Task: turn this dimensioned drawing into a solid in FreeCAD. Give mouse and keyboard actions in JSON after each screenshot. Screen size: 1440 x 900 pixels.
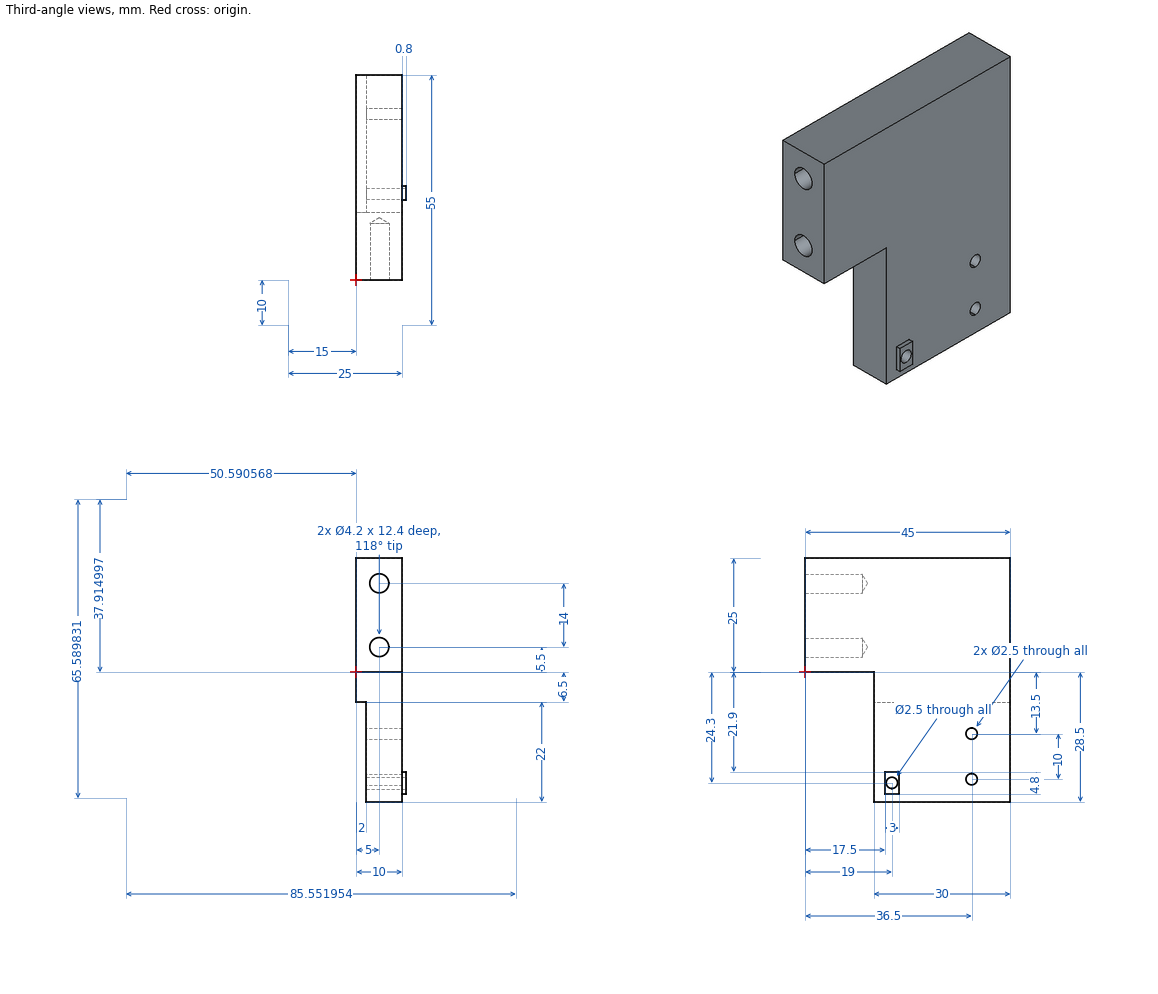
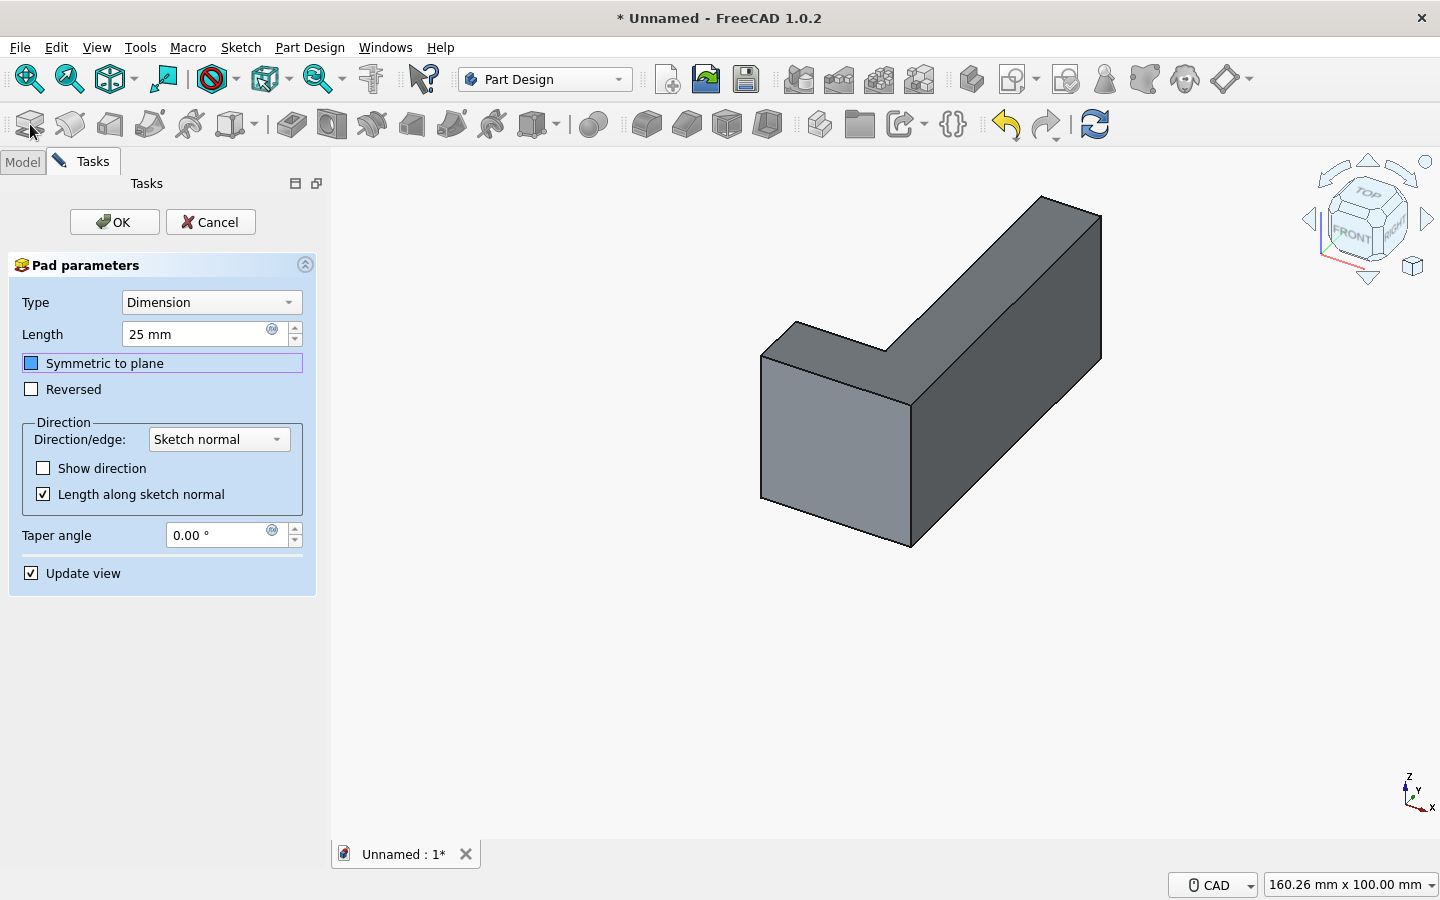
{"action": "left_click", "coordinate": [115, 222]}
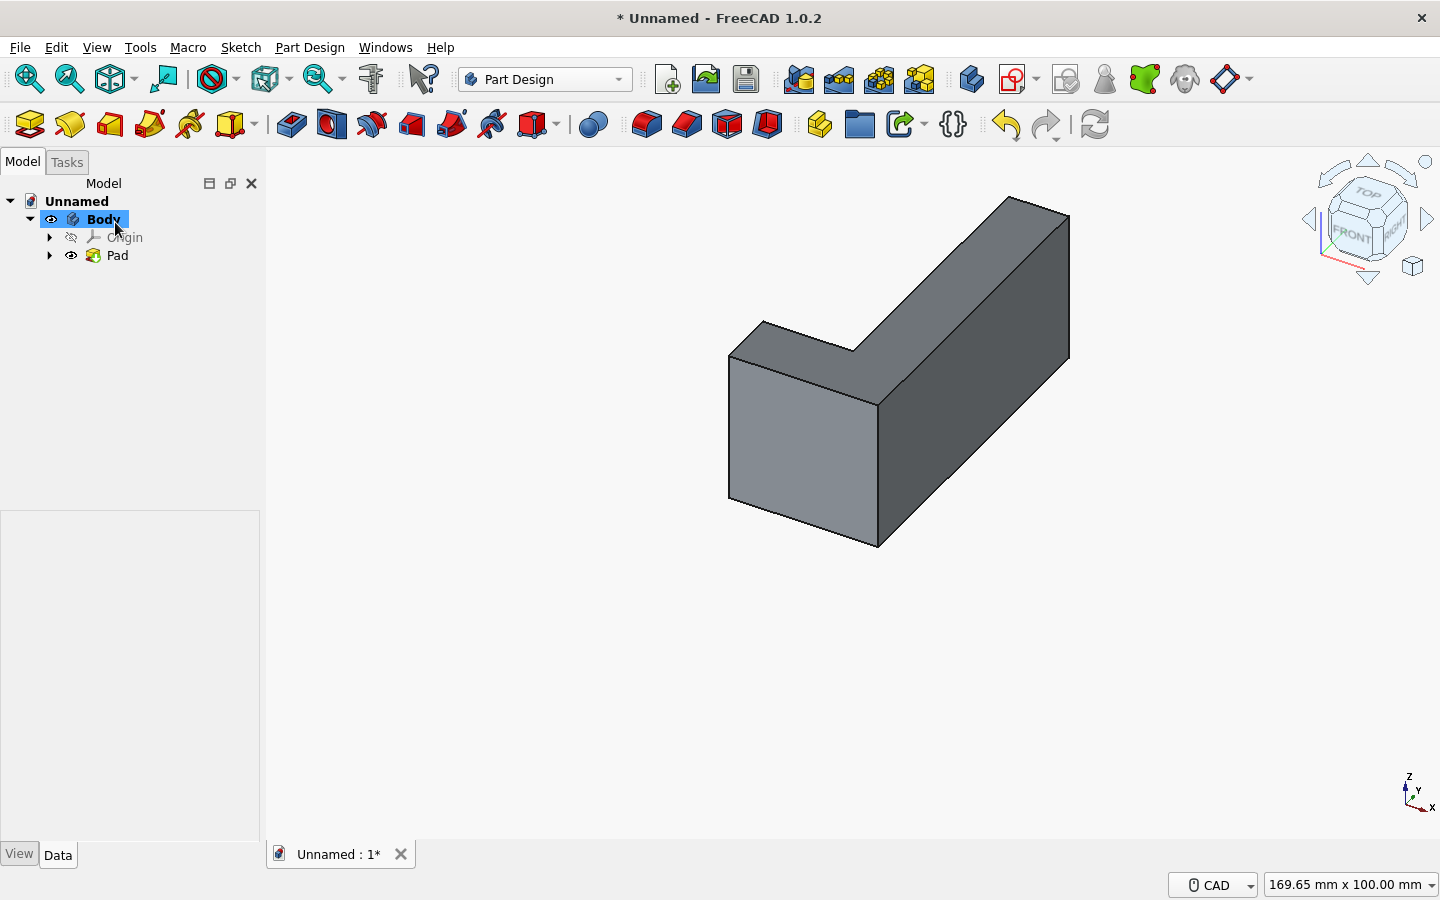
{"action": "key", "text": "6"}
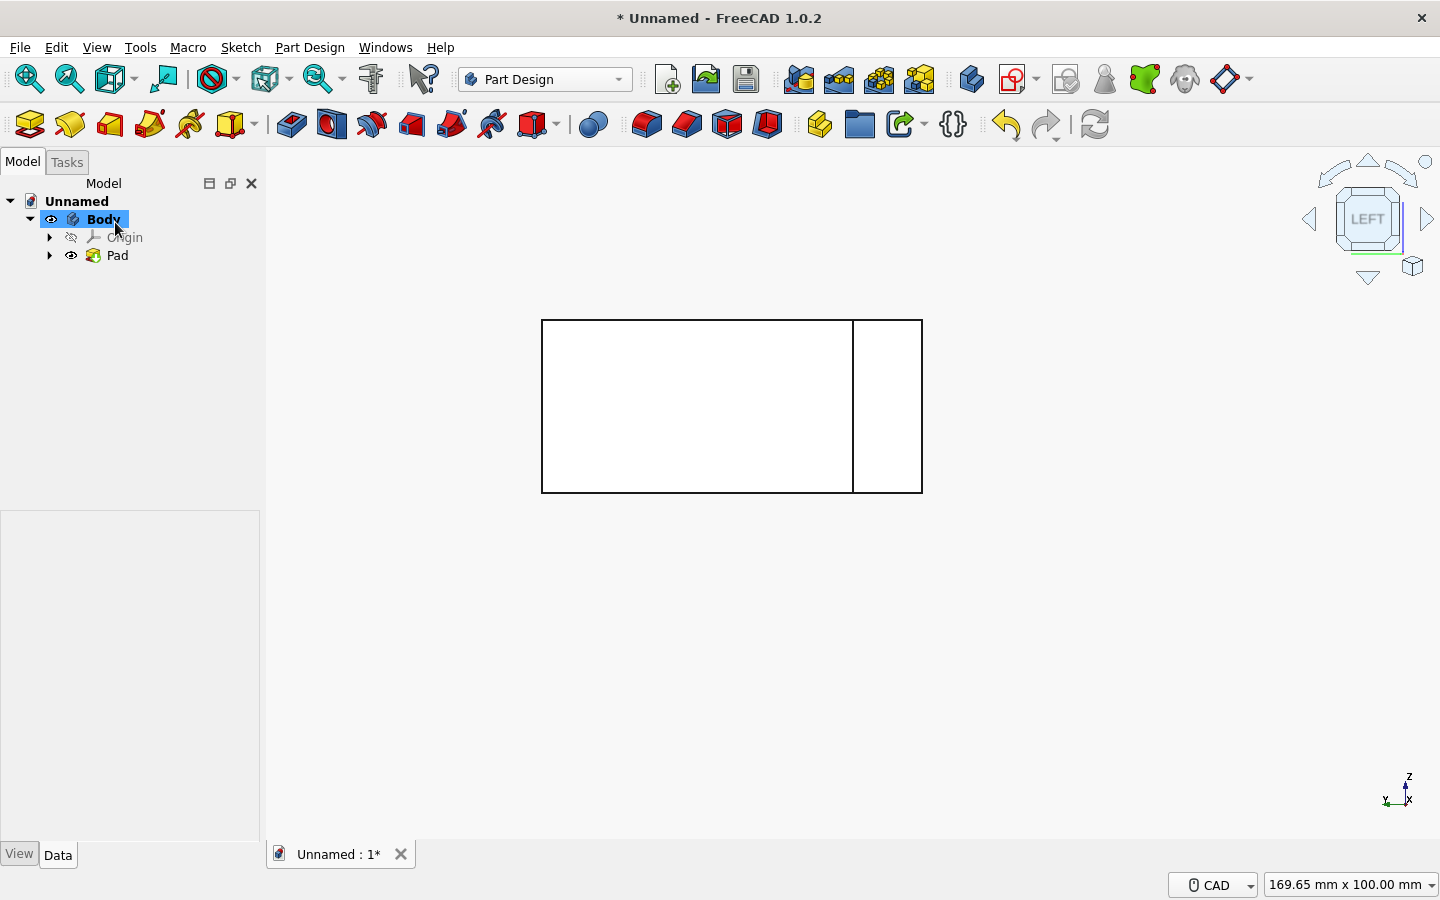
{"action": "key", "text": "v f"}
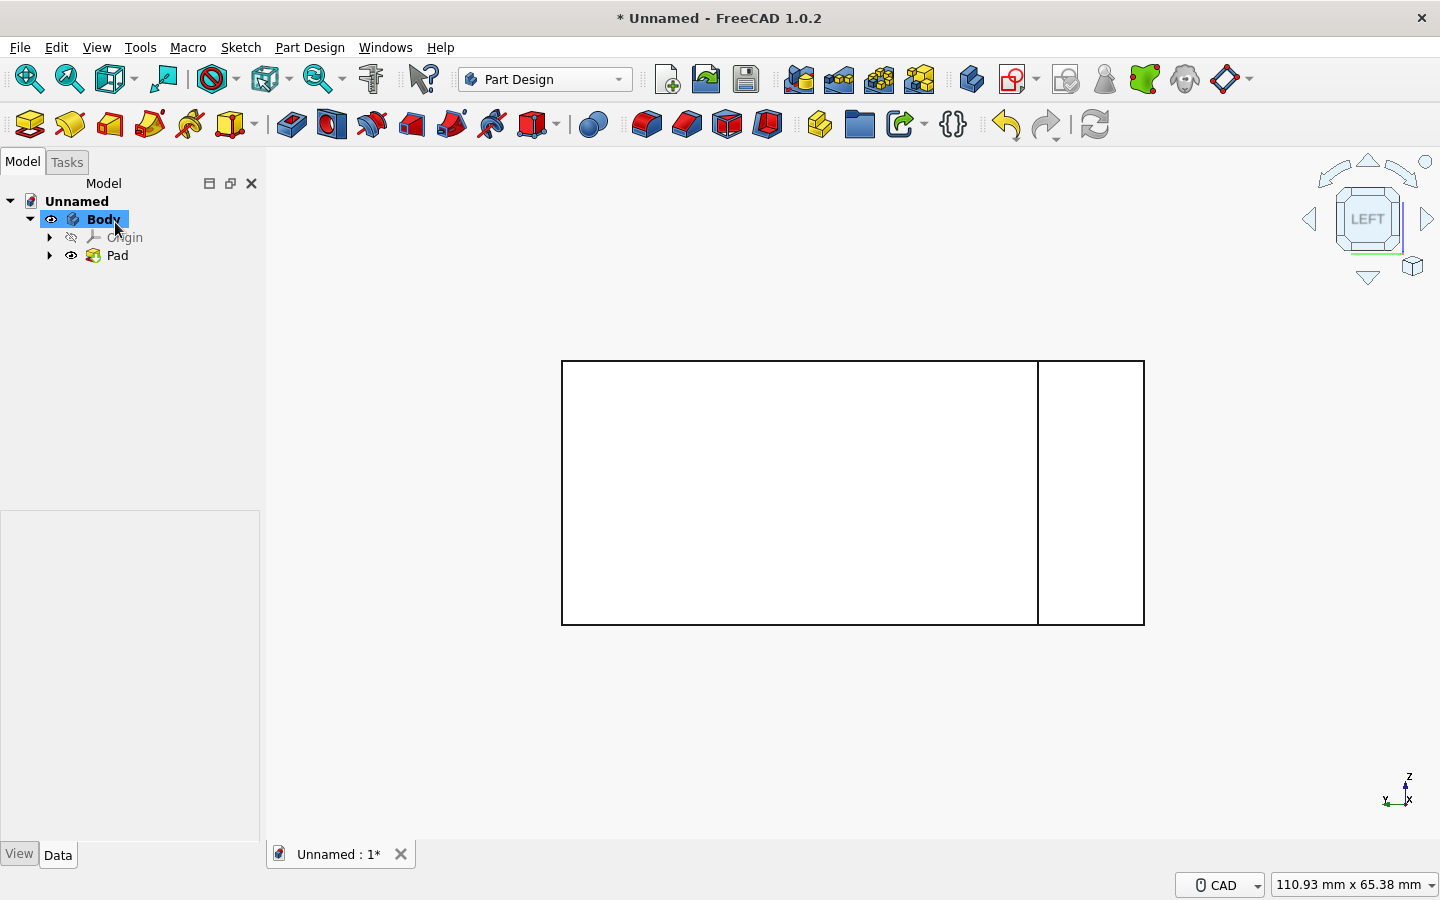
{"action": "left_click", "coordinate": [732, 492]}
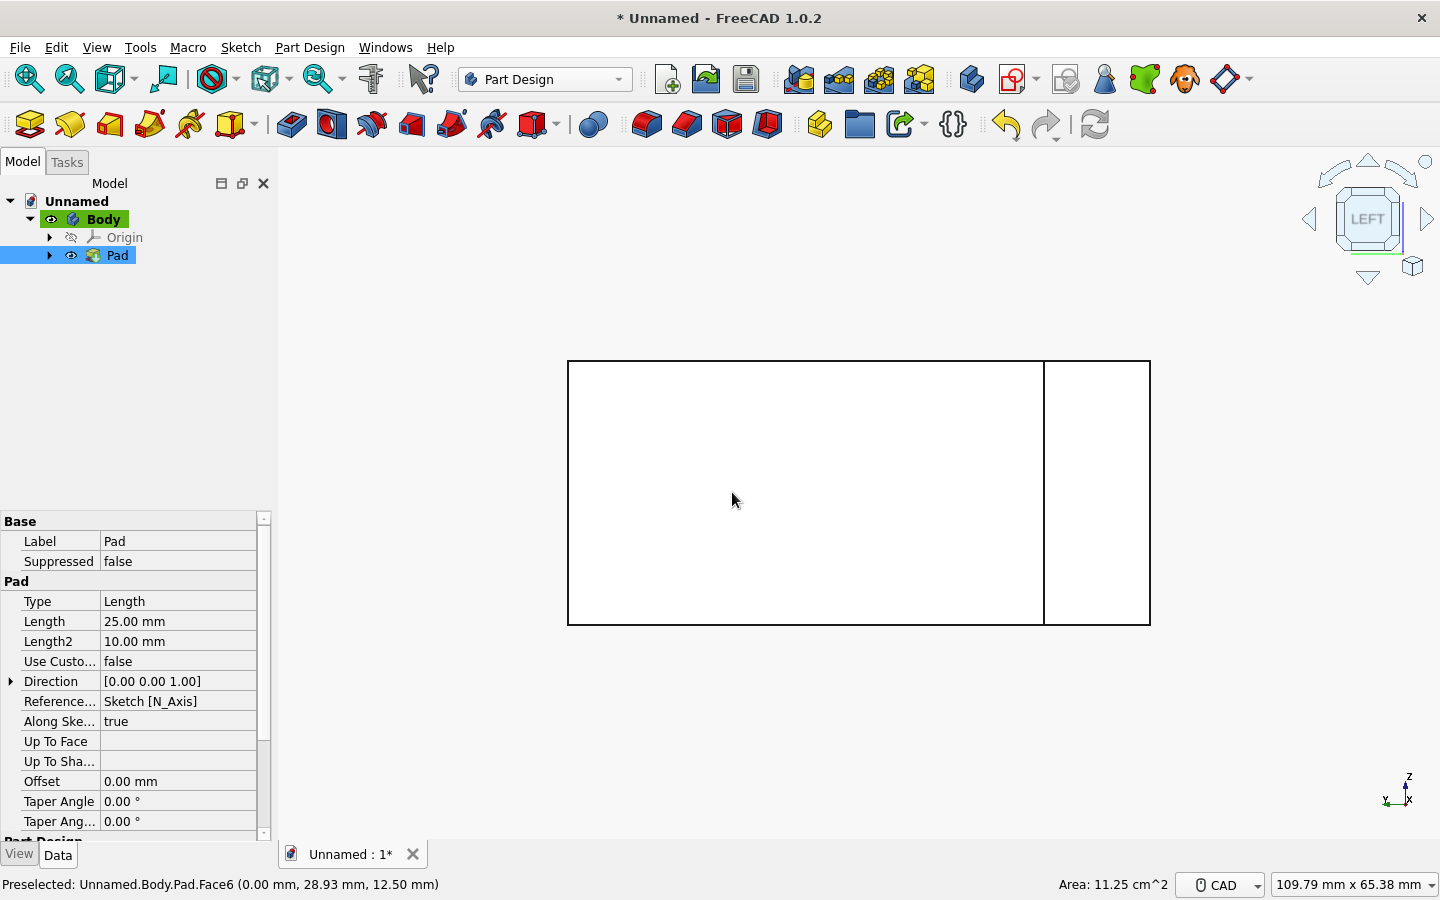
{"action": "left_click", "coordinate": [1012, 80]}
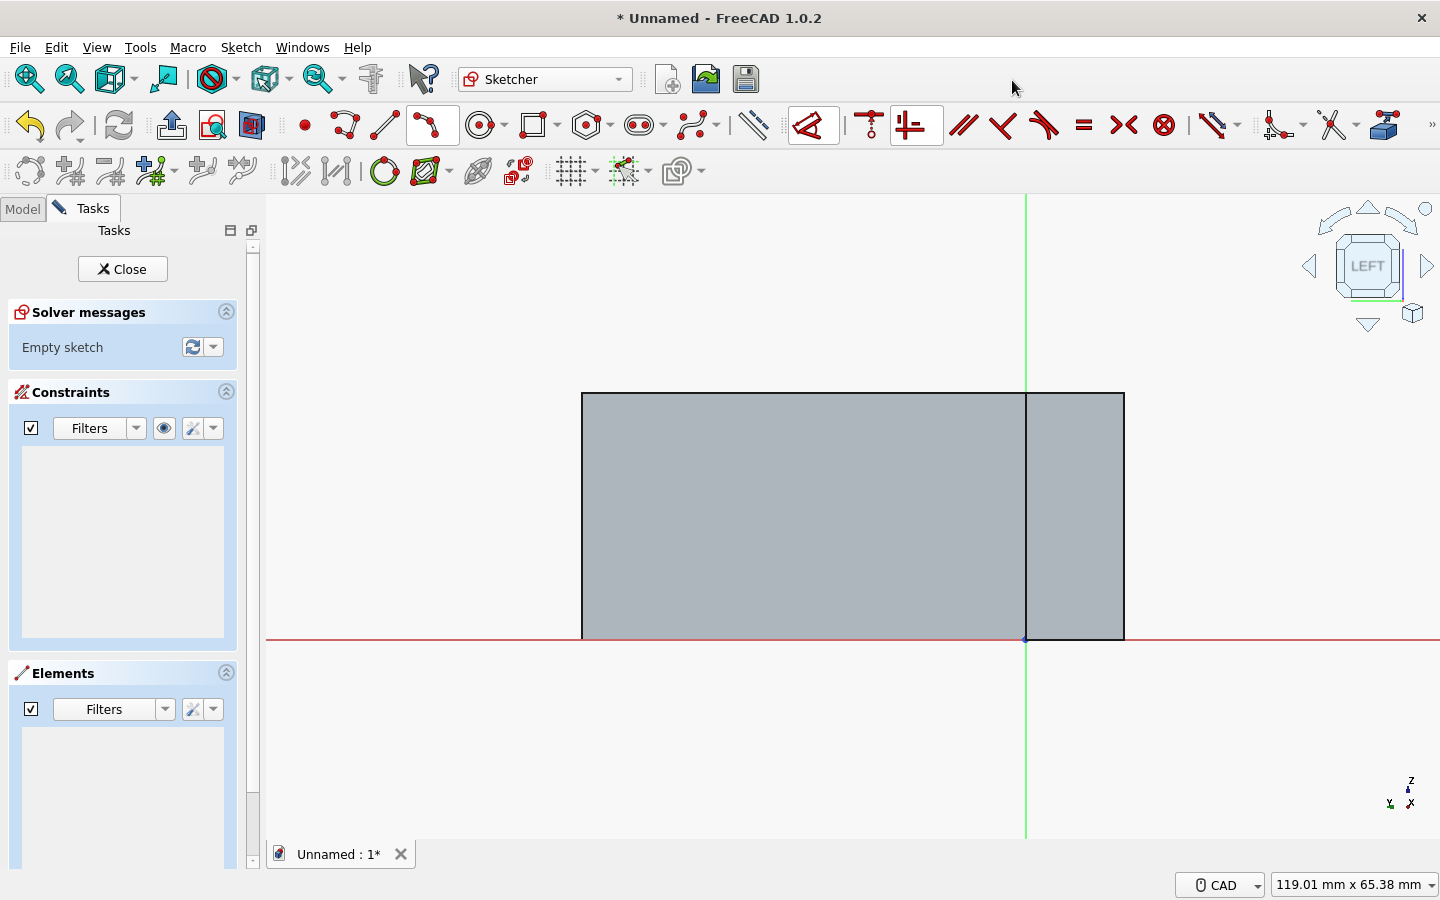
{"action": "scroll", "coordinate": [784, 516], "scroll_direction": "down", "scroll_amount": 5}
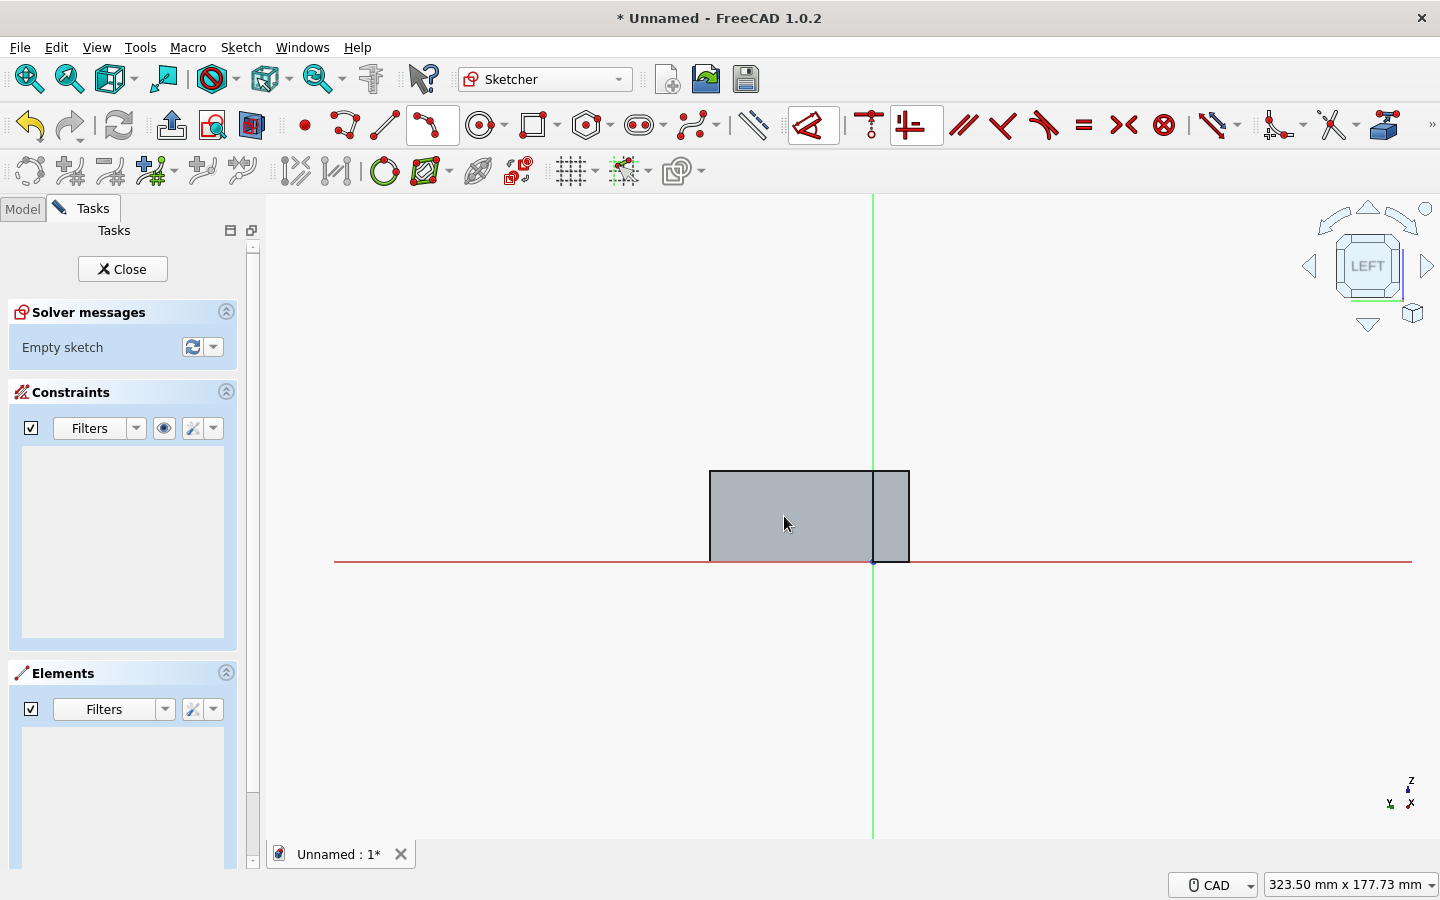
{"action": "scroll", "coordinate": [794, 645], "scroll_direction": "up", "scroll_amount": 7}